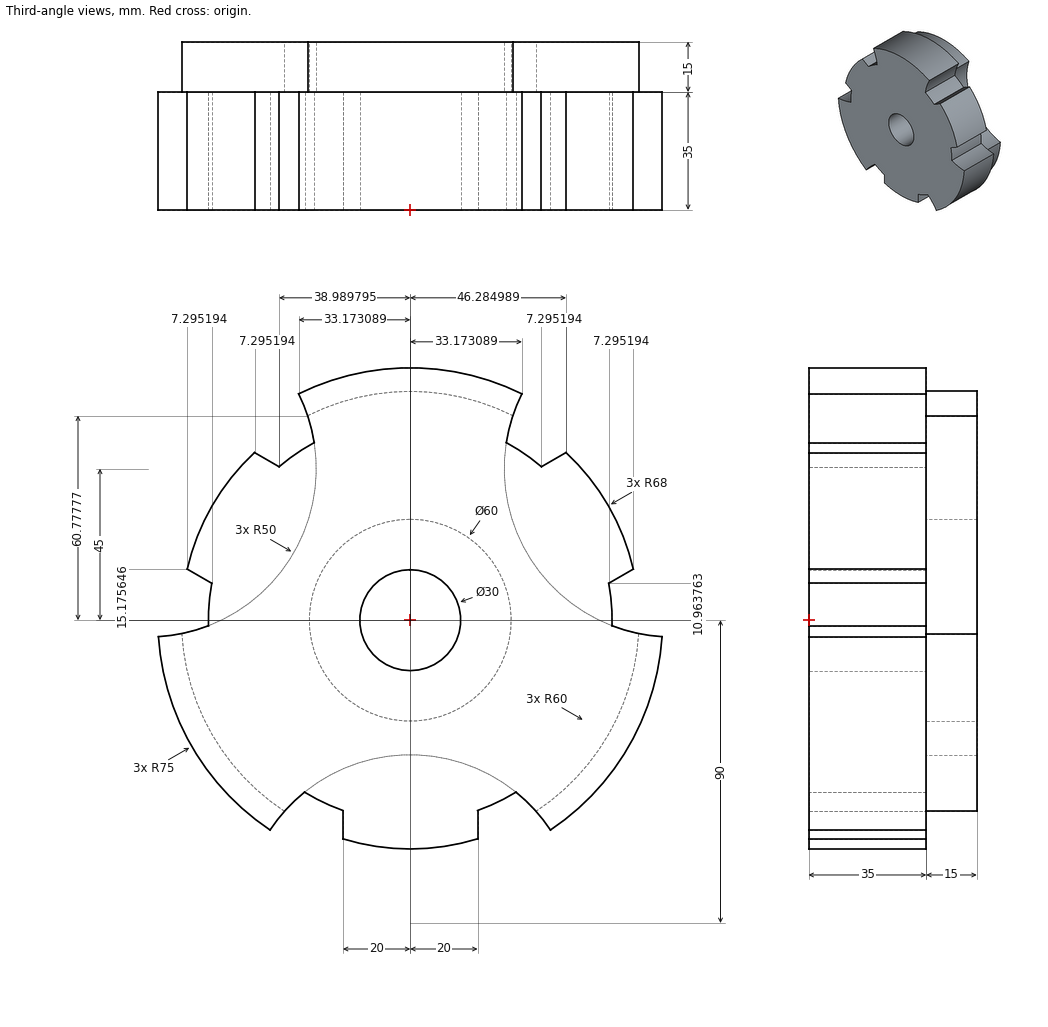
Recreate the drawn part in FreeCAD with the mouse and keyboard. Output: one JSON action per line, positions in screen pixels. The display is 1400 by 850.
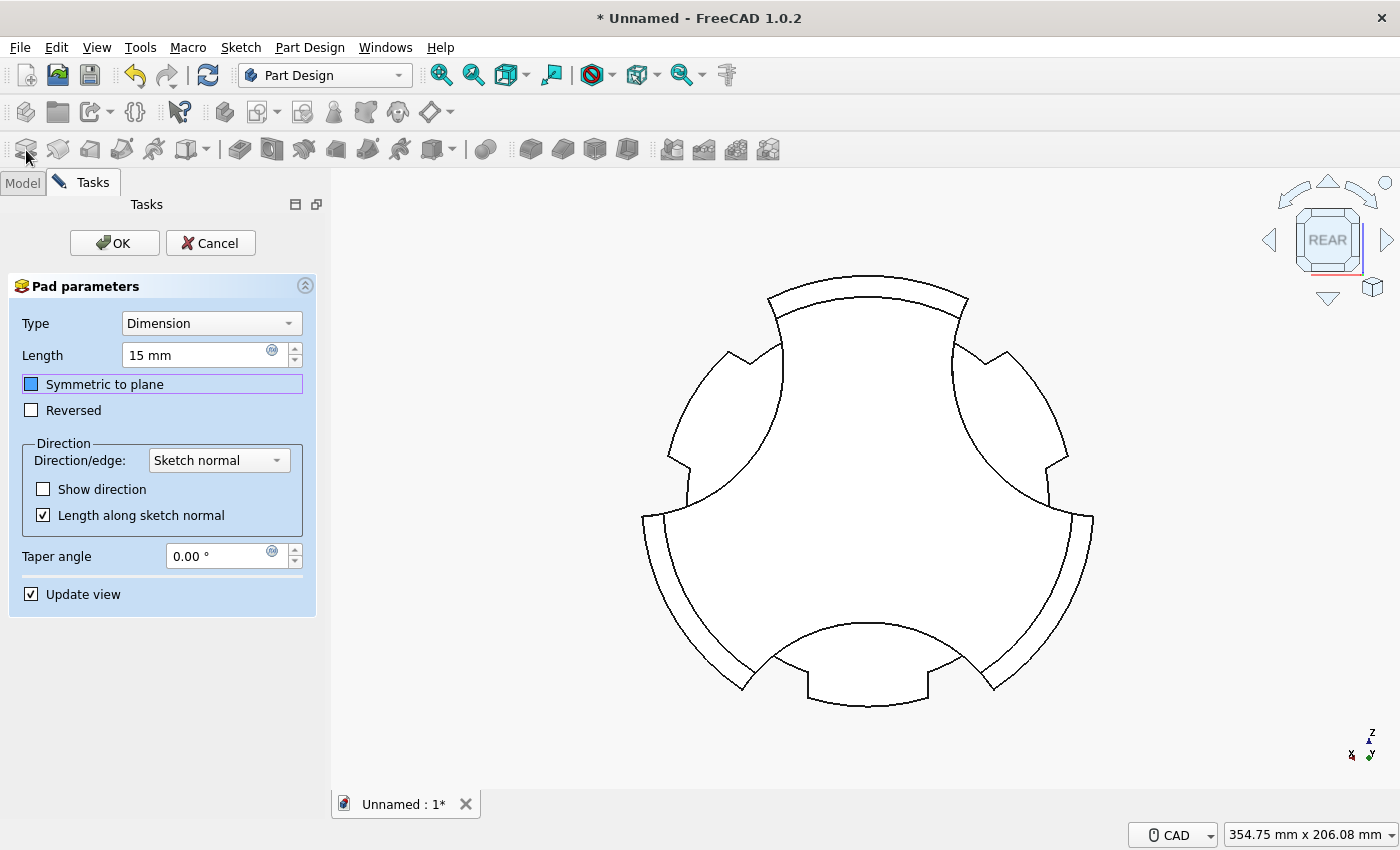
{"action": "left_click", "coordinate": [115, 243]}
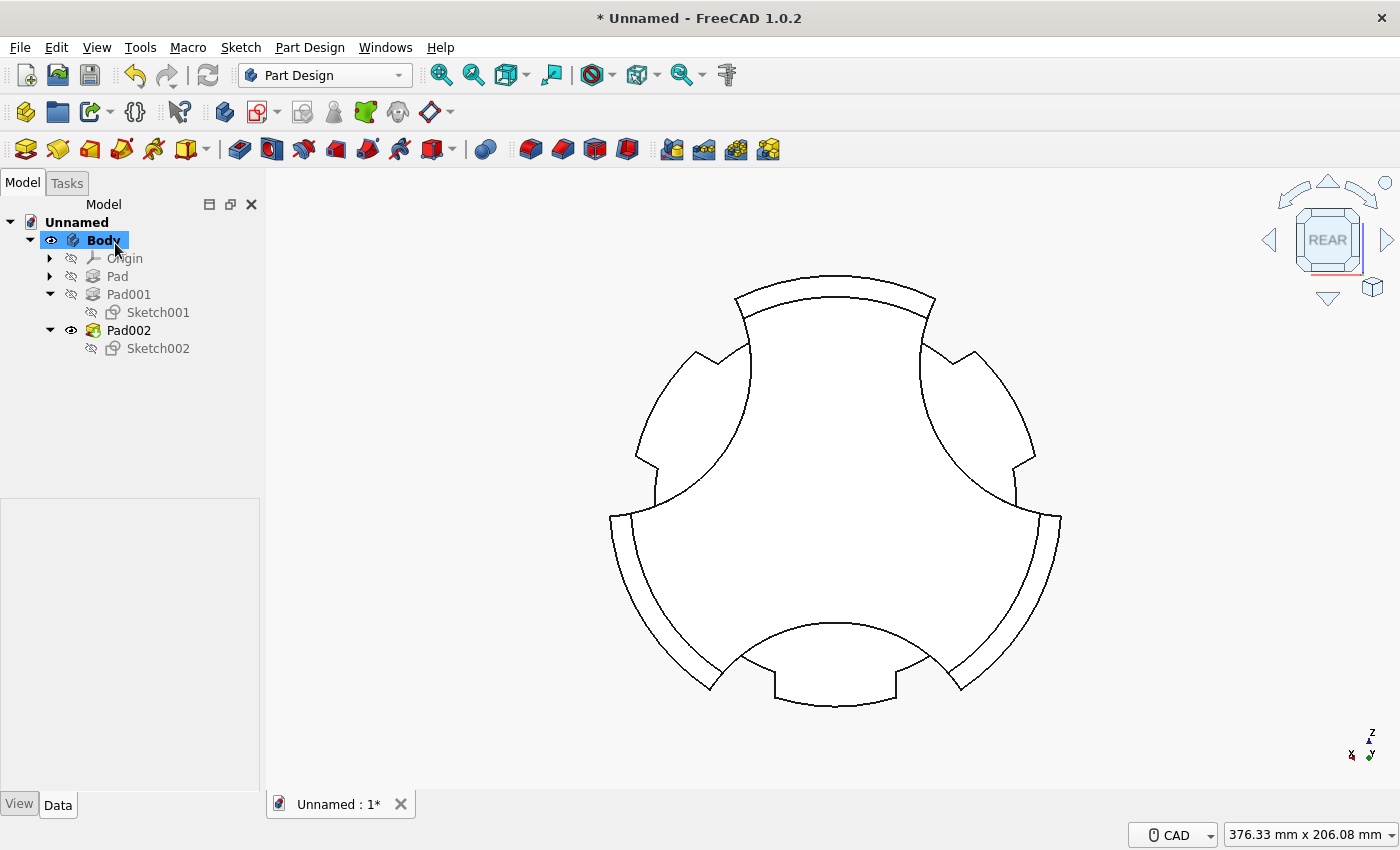
{"action": "left_click", "coordinate": [835, 484]}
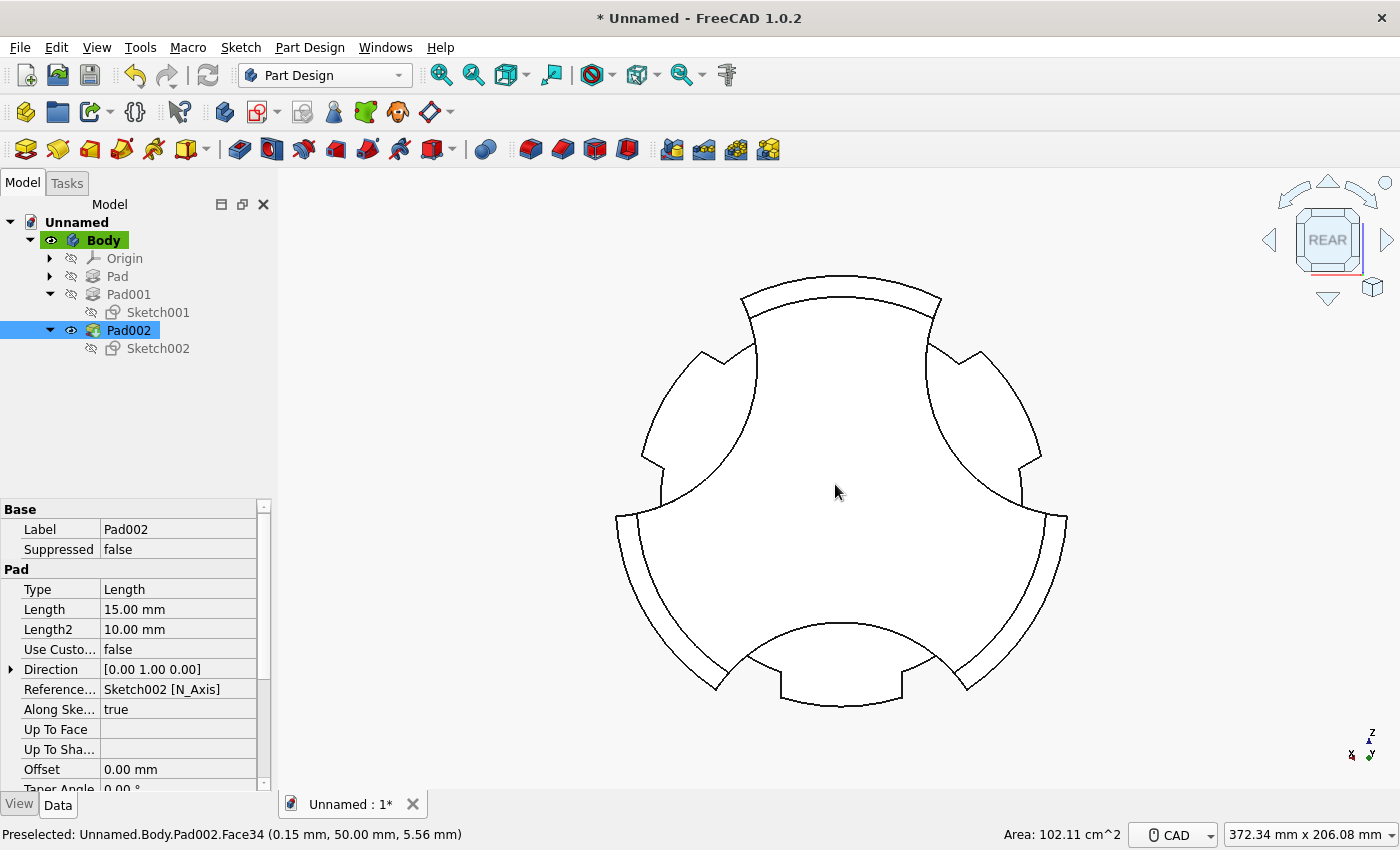
{"action": "left_click", "coordinate": [258, 112]}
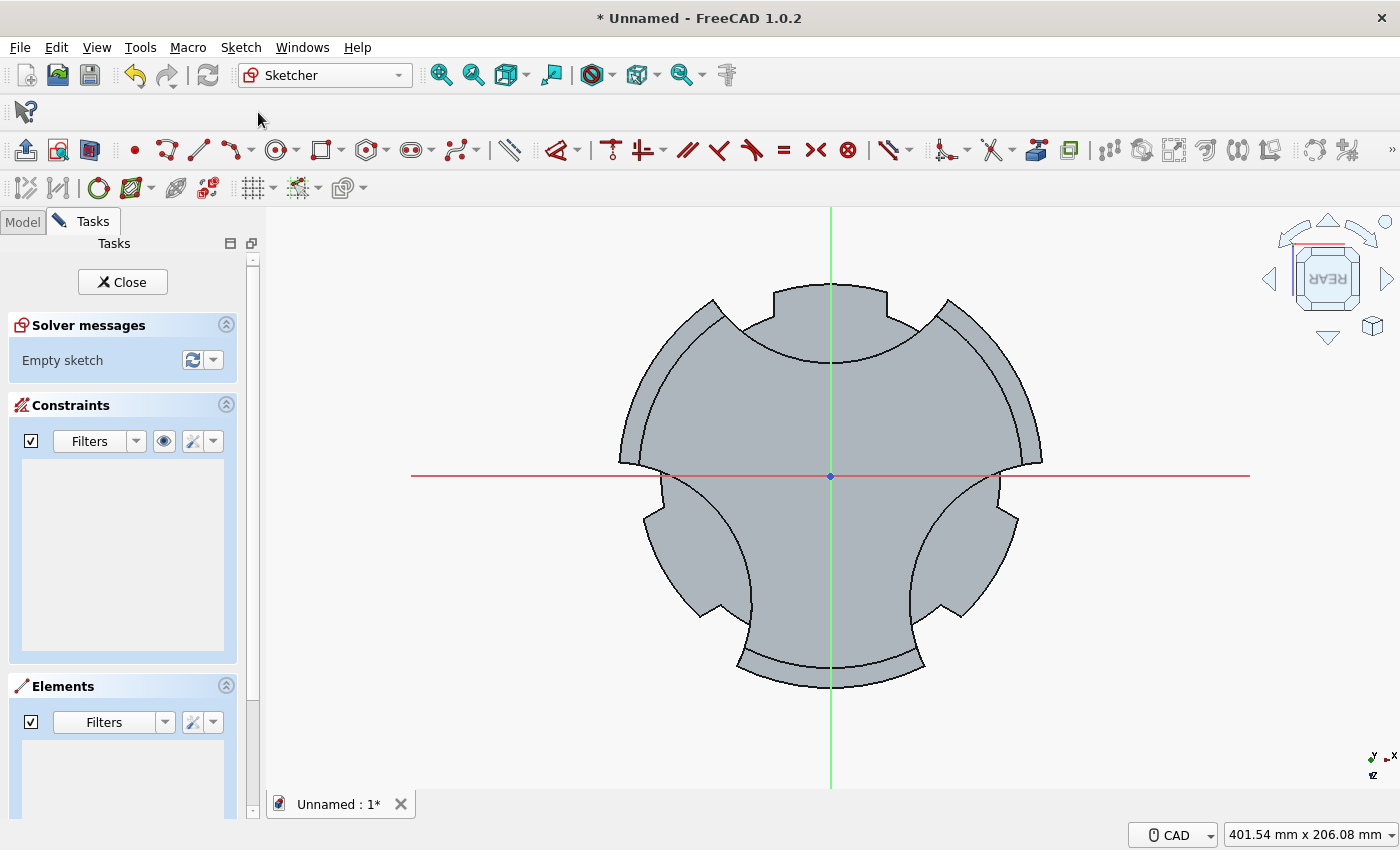
{"action": "scroll", "coordinate": [885, 458], "scroll_direction": "up", "scroll_amount": 4}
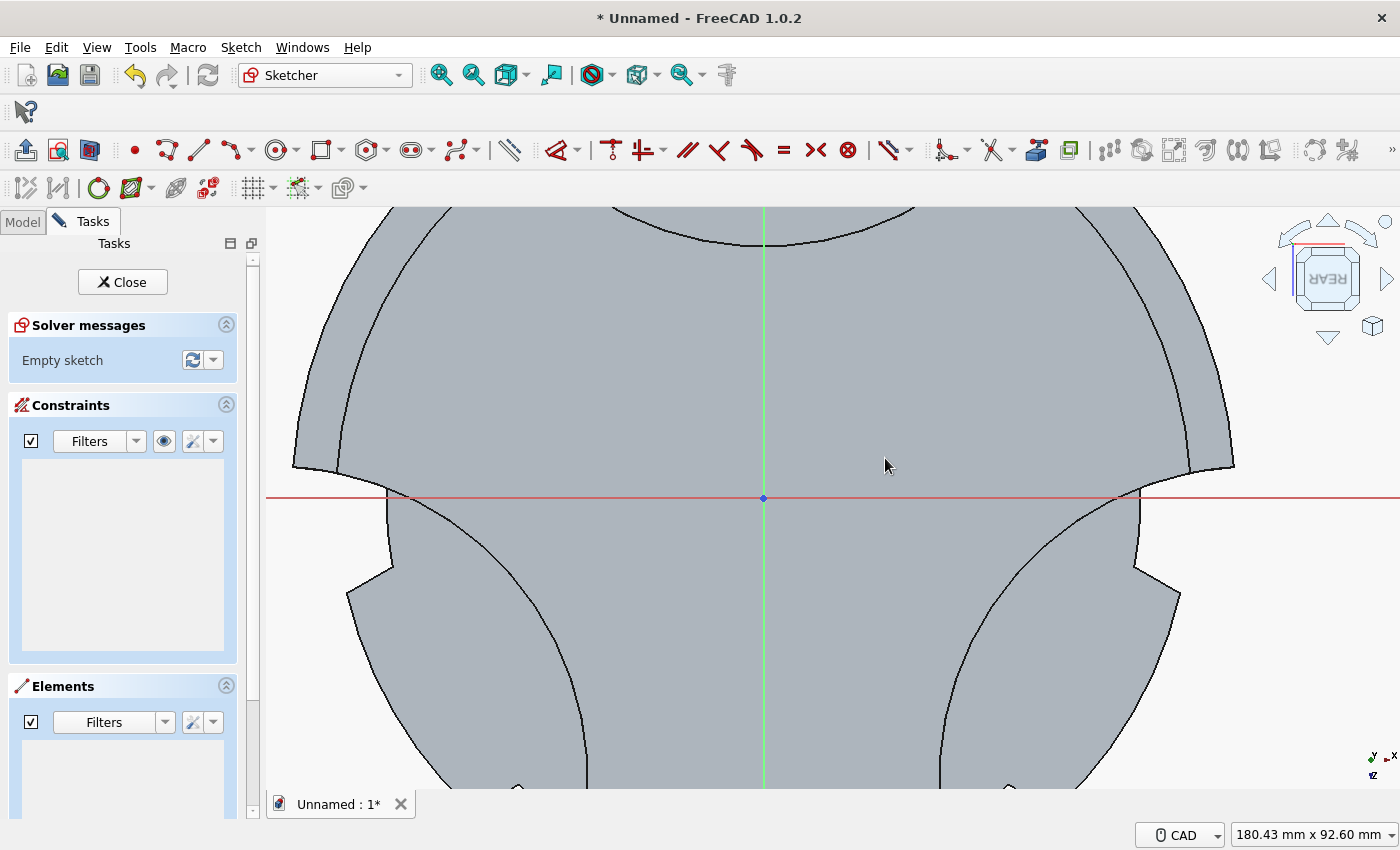
{"action": "left_click", "coordinate": [276, 150]}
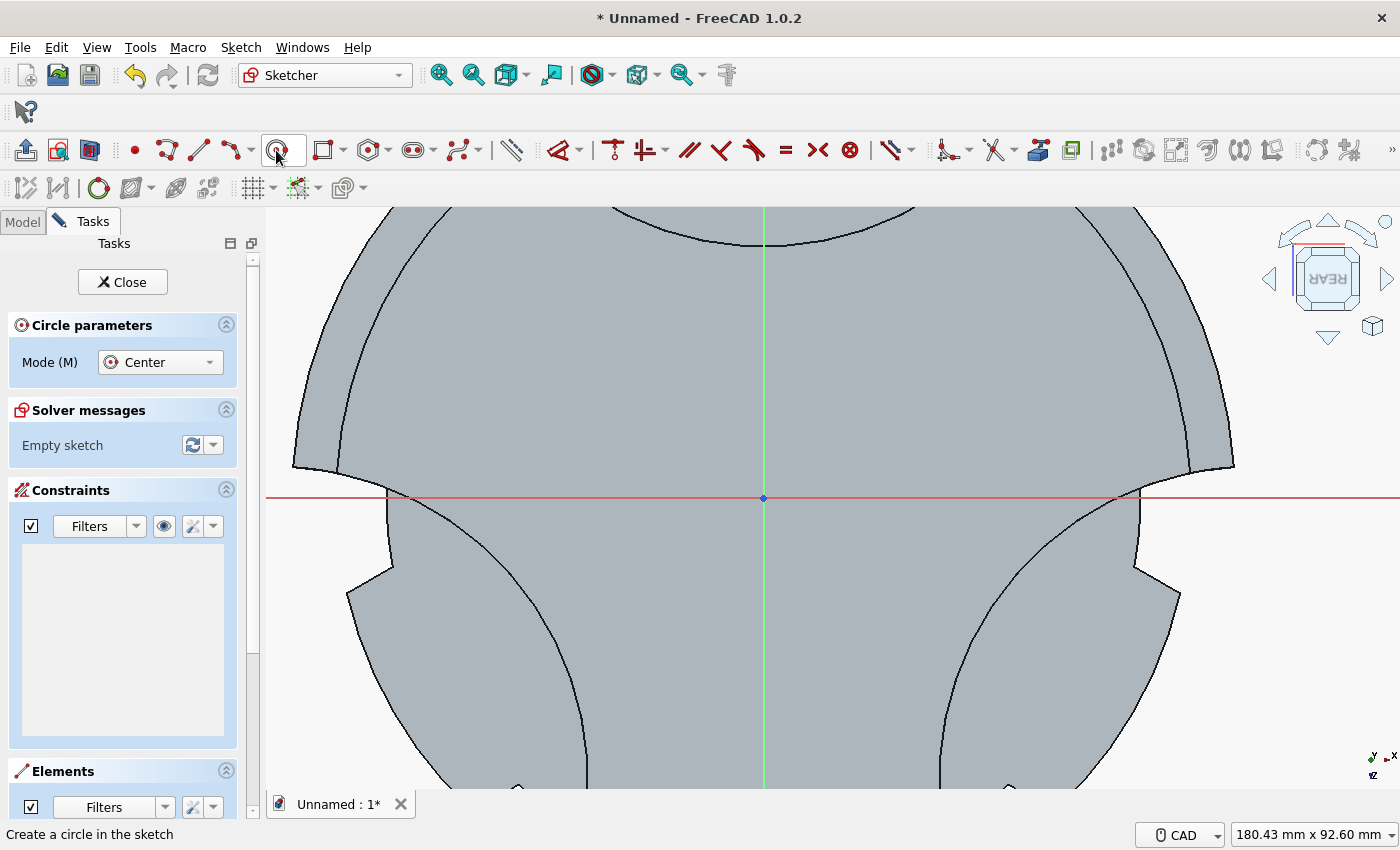
{"action": "left_click", "coordinate": [764, 498]}
{"action": "left_click", "coordinate": [897, 365]}
{"action": "key", "text": "Escape"}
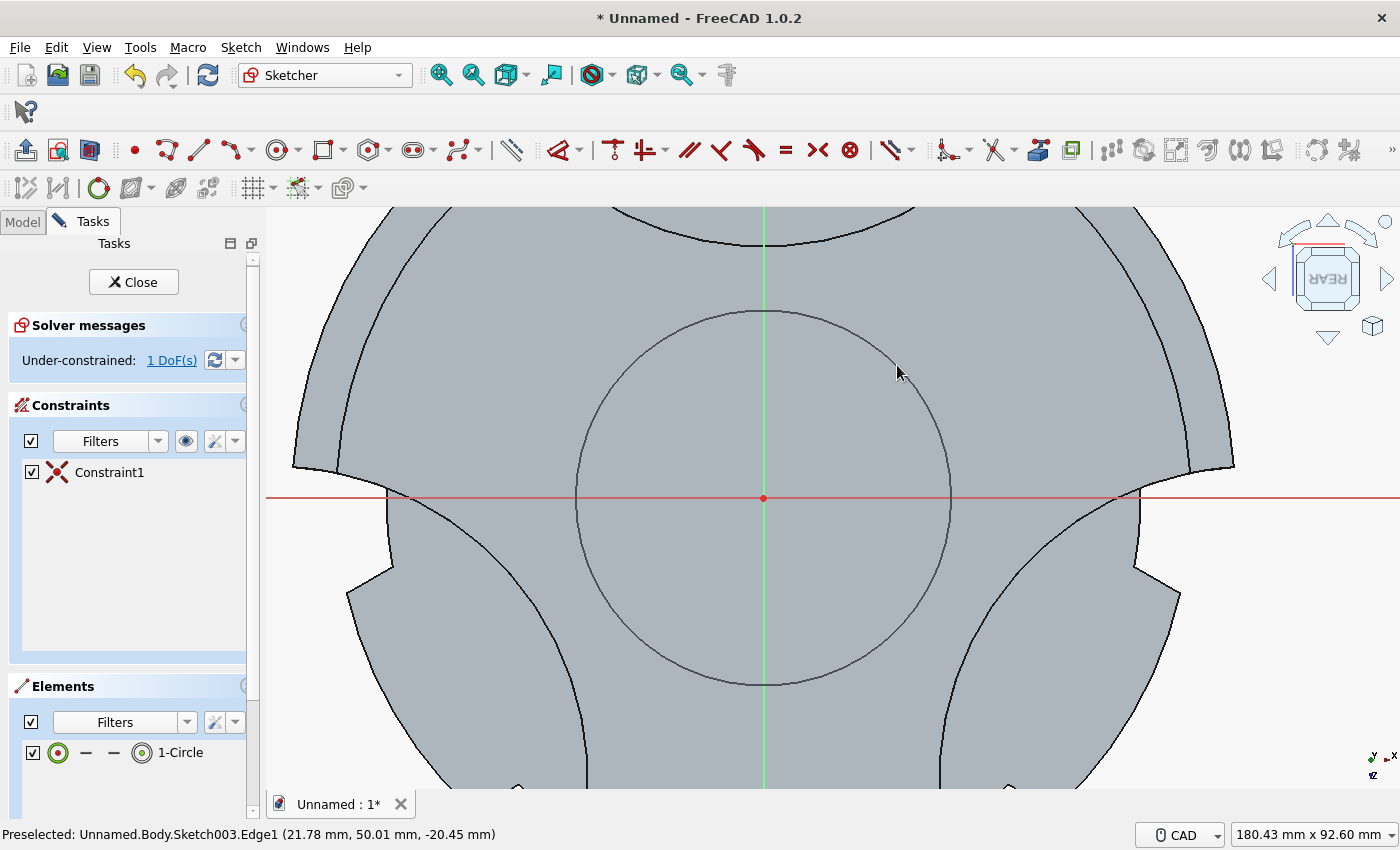
{"action": "left_click", "coordinate": [558, 150]}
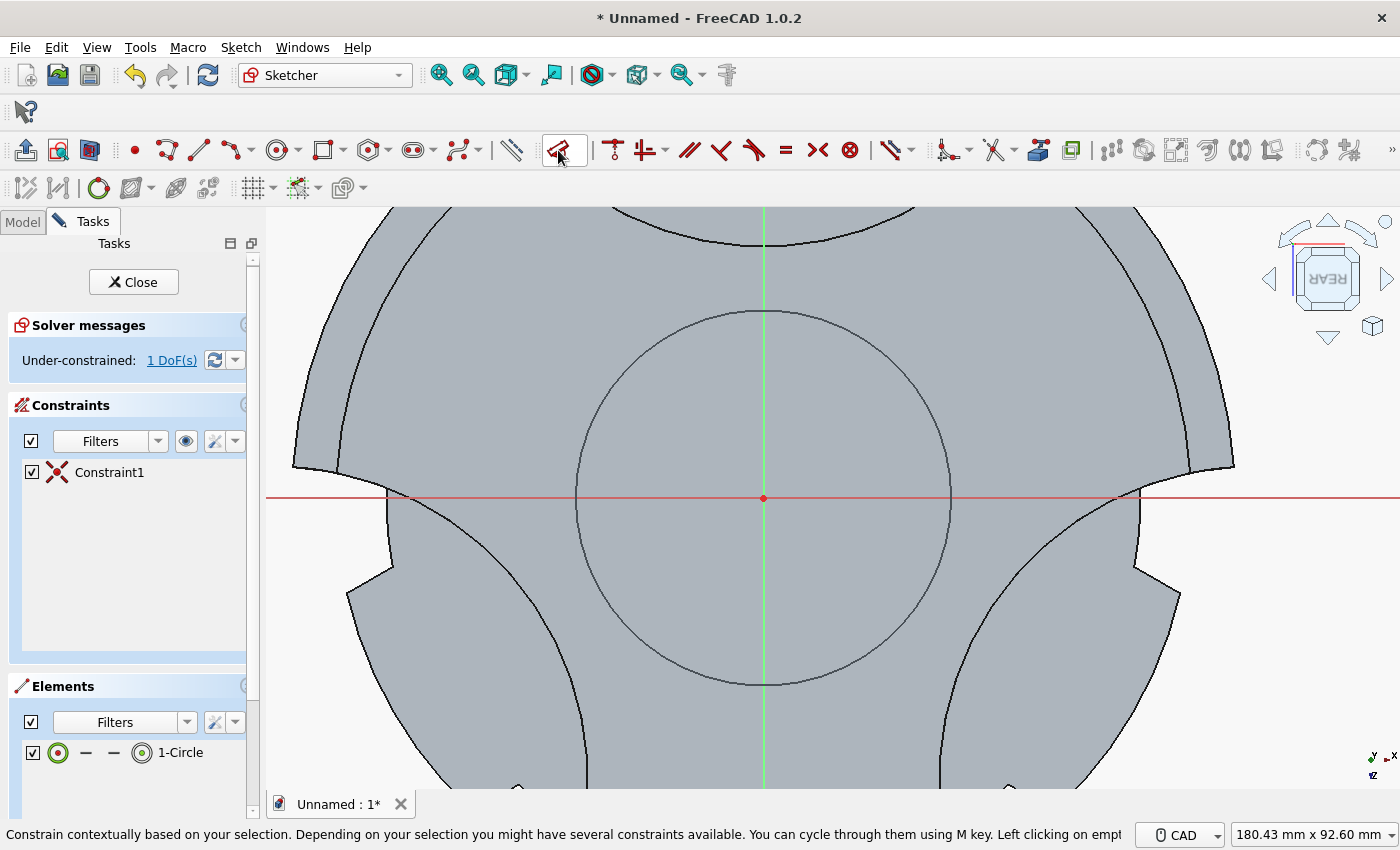
{"action": "left_click", "coordinate": [896, 365]}
{"action": "left_click", "coordinate": [919, 342]}